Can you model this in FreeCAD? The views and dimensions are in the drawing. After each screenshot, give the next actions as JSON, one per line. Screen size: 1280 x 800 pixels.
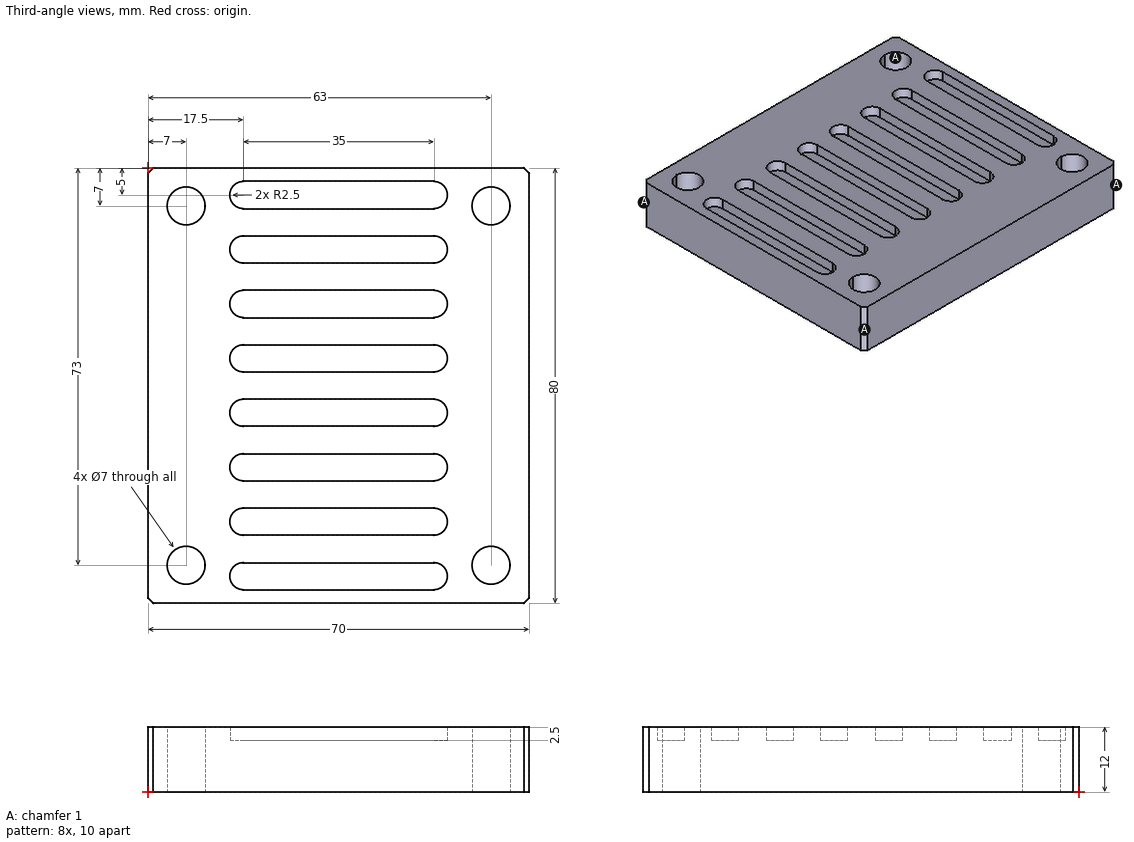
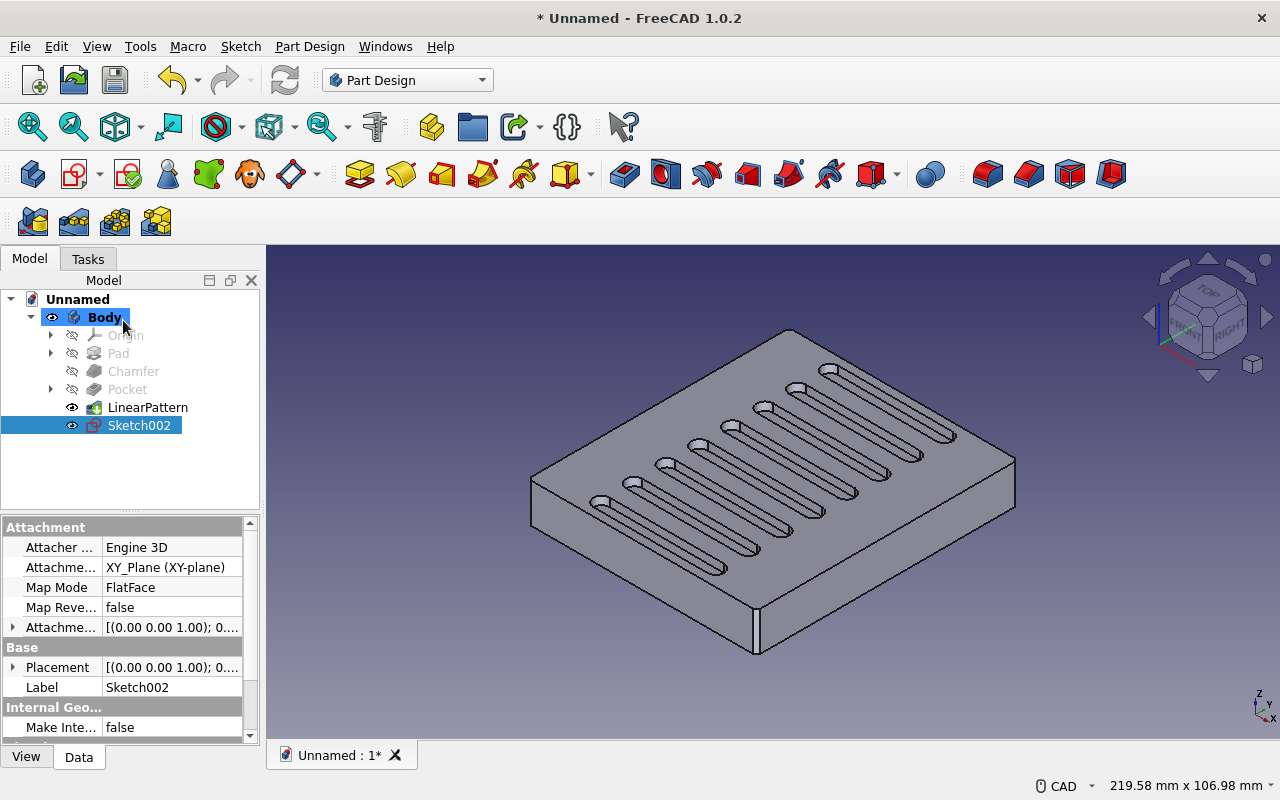
{"action": "left_click", "coordinate": [666, 174]}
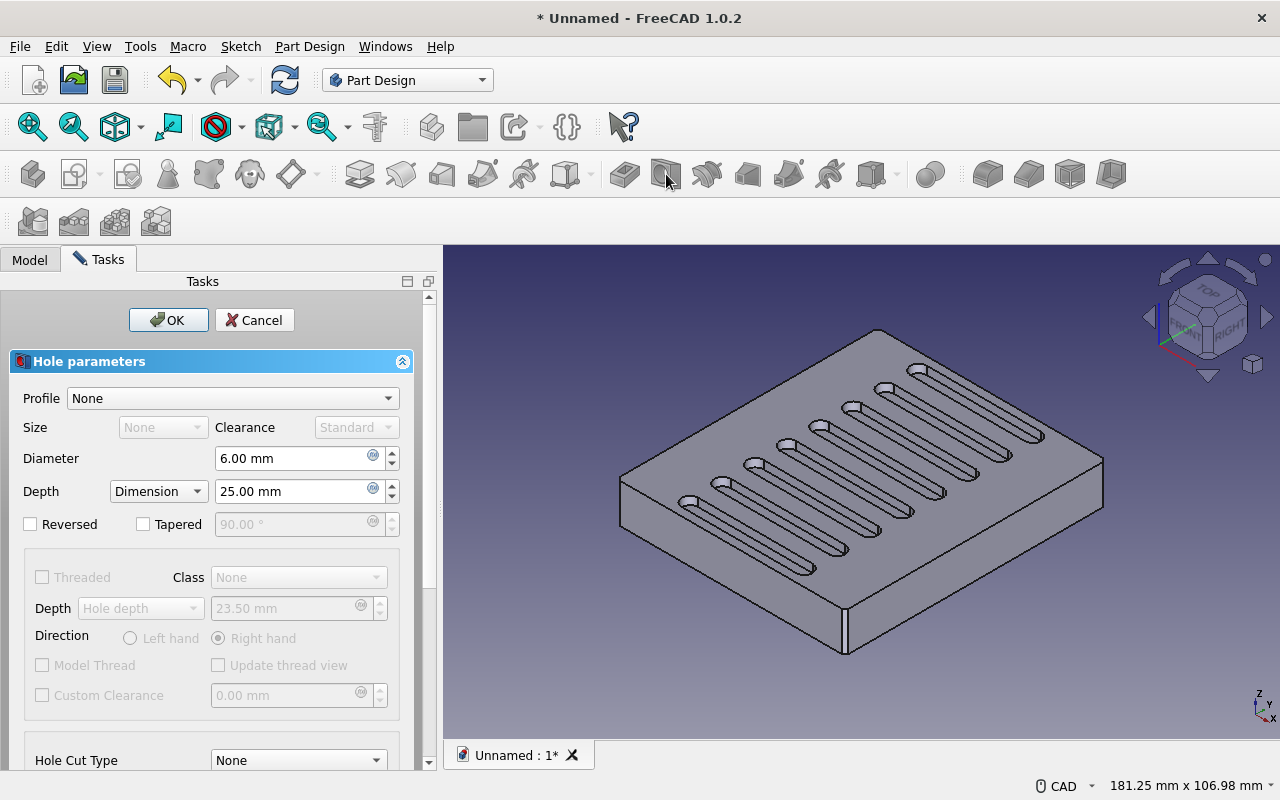
{"action": "triple_click", "coordinate": [300, 458]}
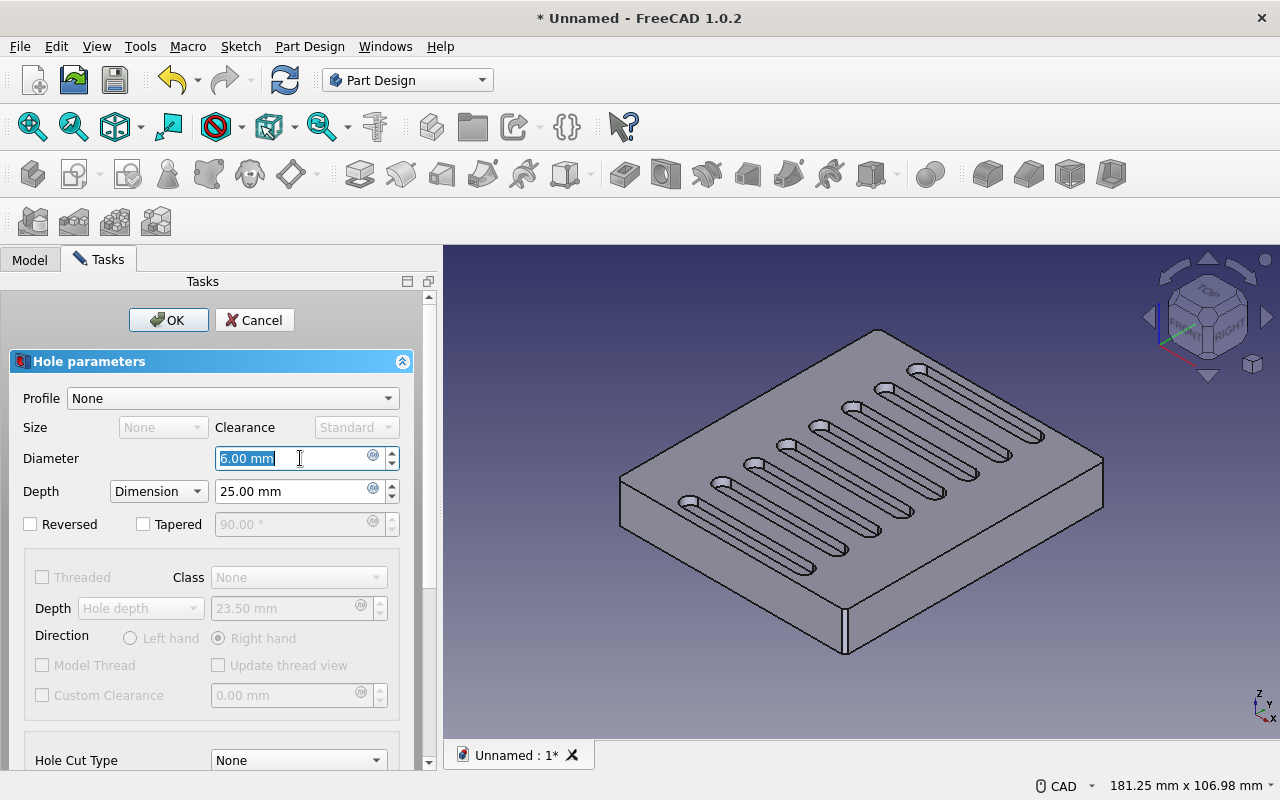
{"action": "type", "text": "7"}
{"action": "key", "text": "Tab"}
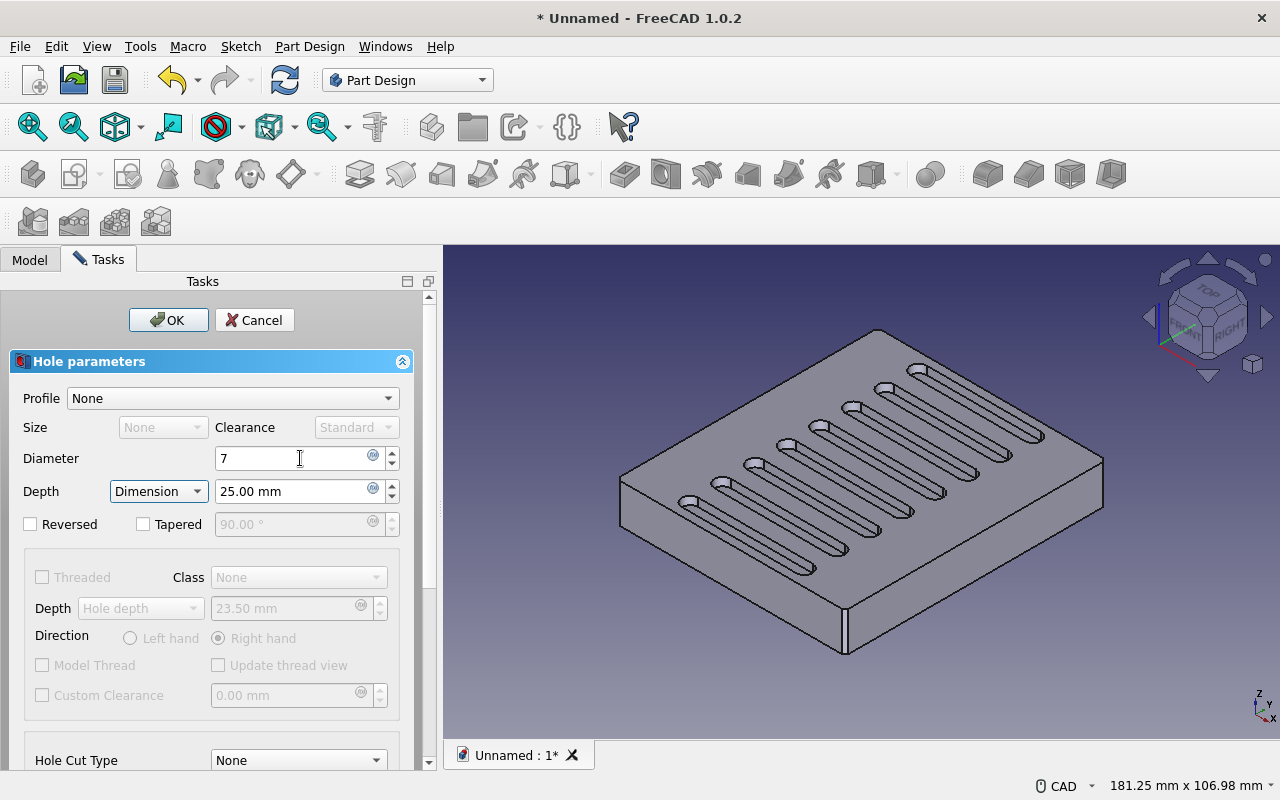
{"action": "left_click", "coordinate": [160, 492]}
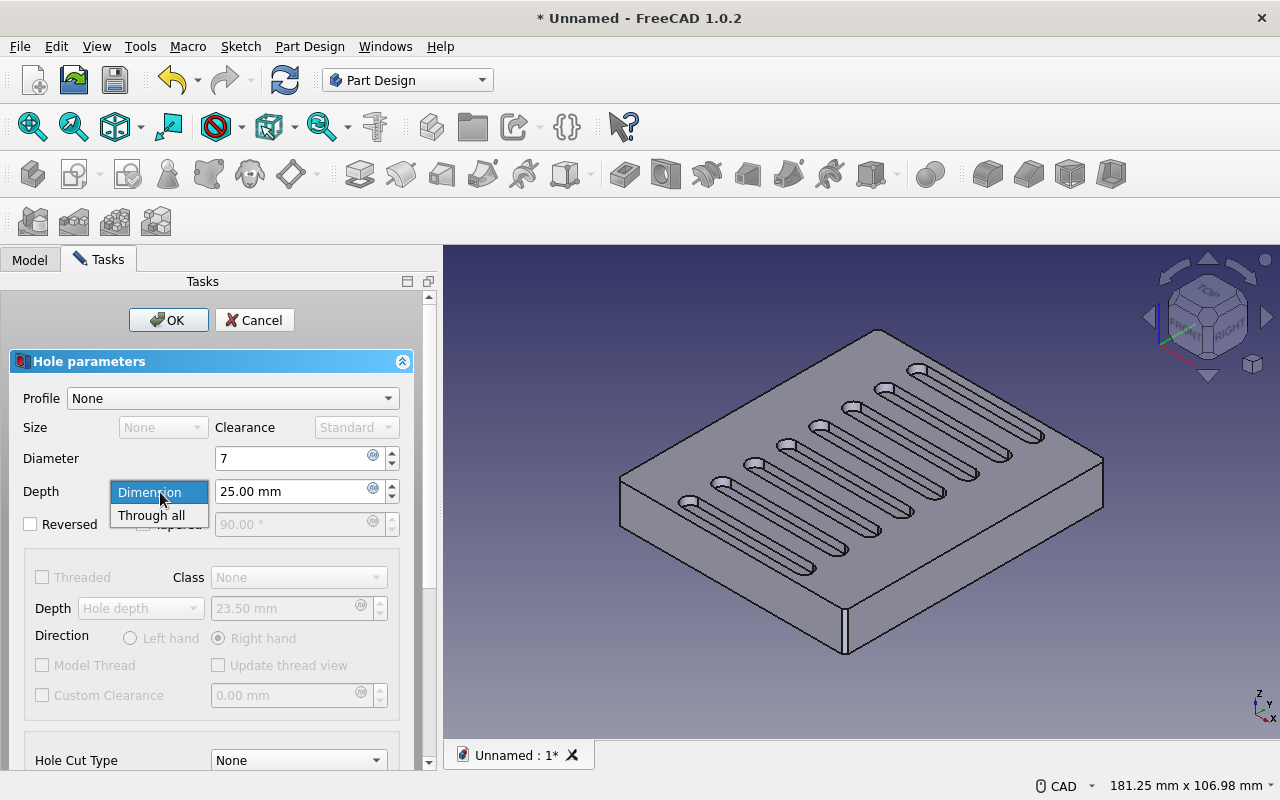
{"action": "left_click", "coordinate": [158, 516]}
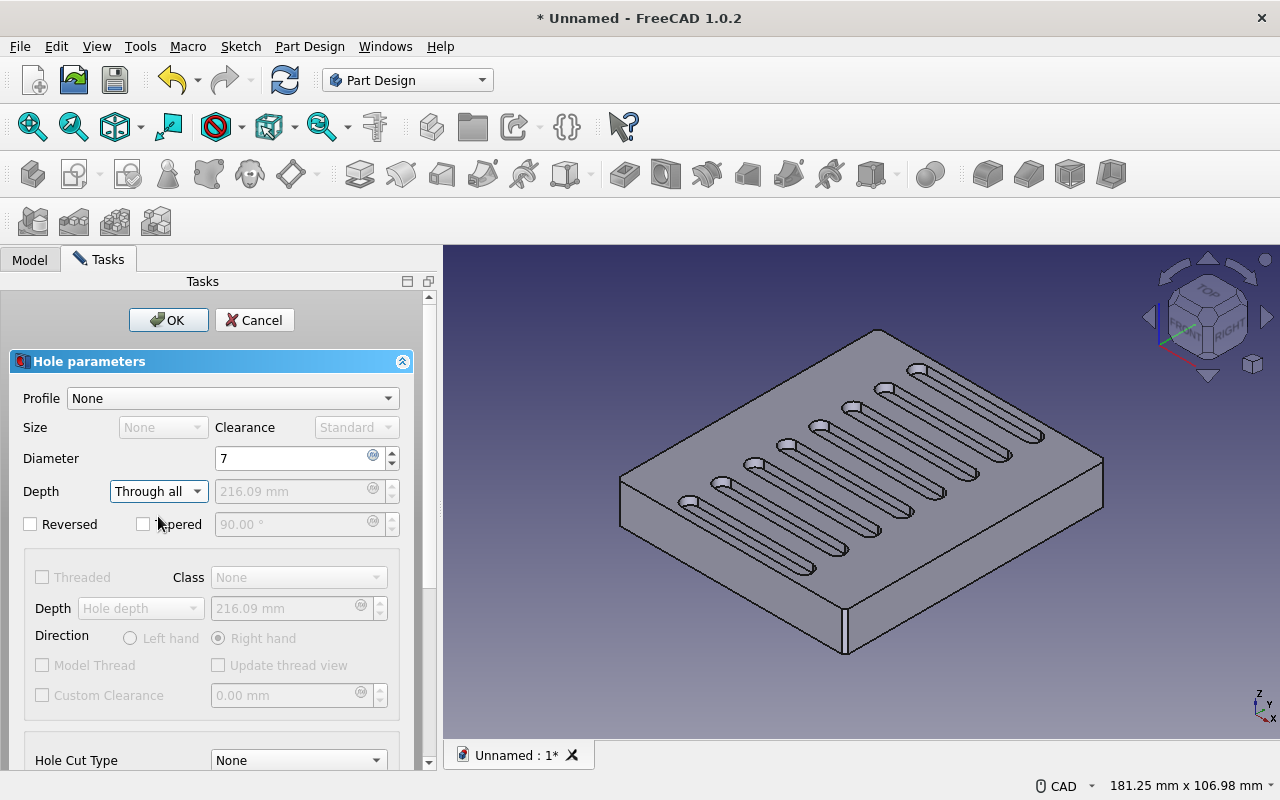
{"action": "left_click", "coordinate": [31, 524]}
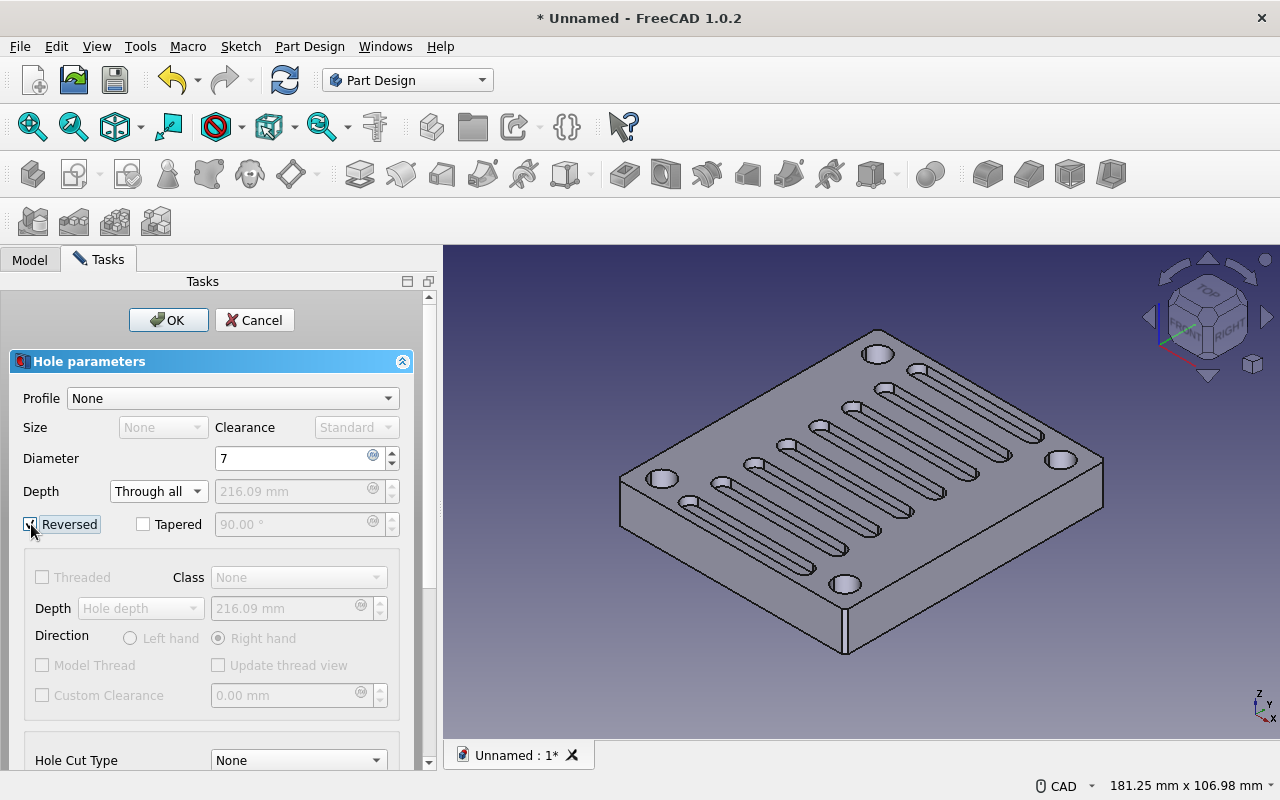
{"action": "left_click", "coordinate": [169, 320]}